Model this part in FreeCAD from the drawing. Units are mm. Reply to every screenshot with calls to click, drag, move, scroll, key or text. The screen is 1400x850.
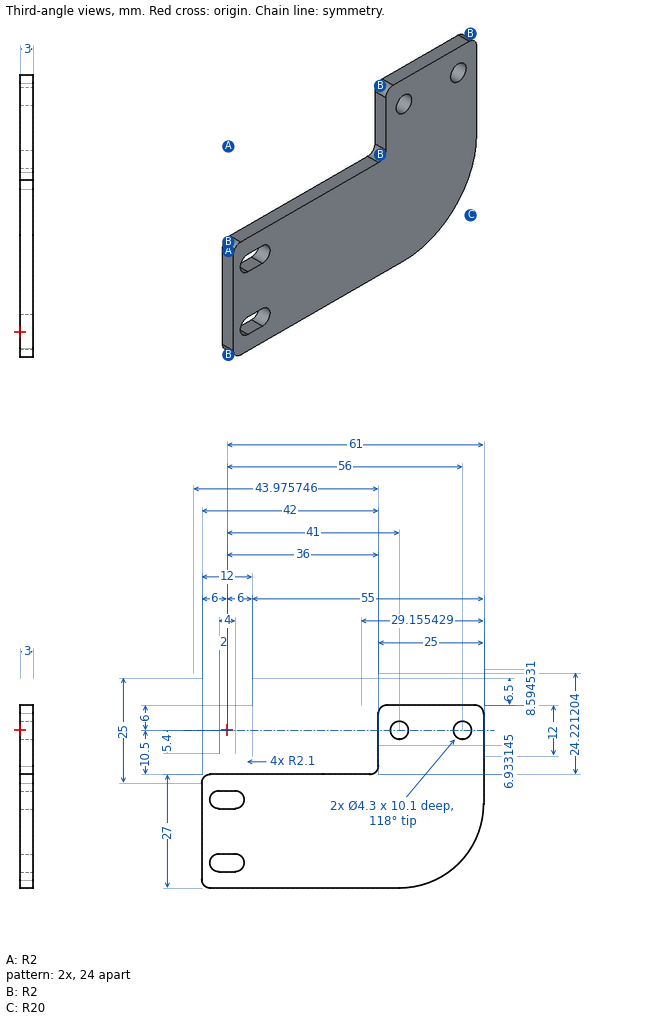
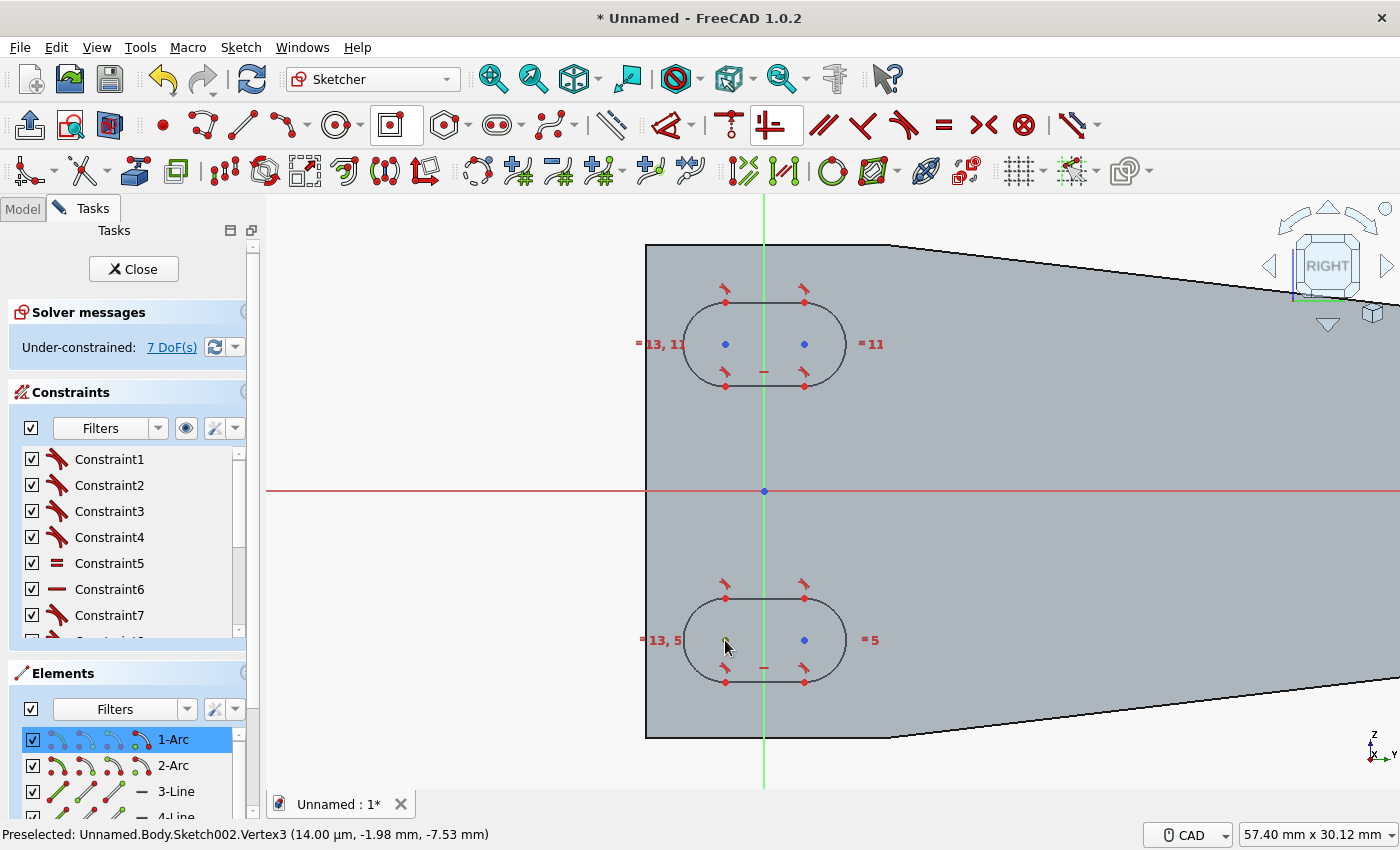
click(725, 345)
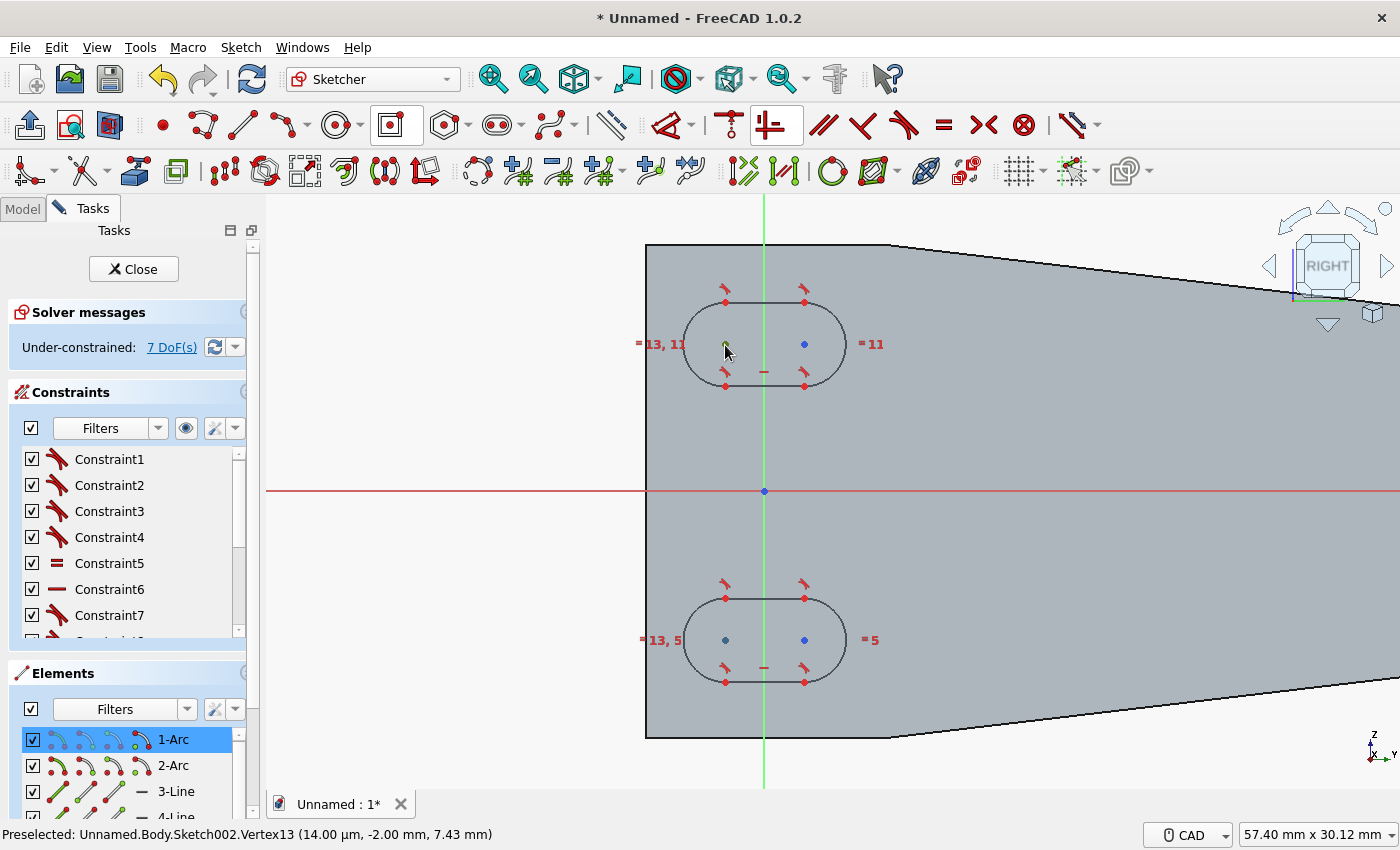
click(361, 491)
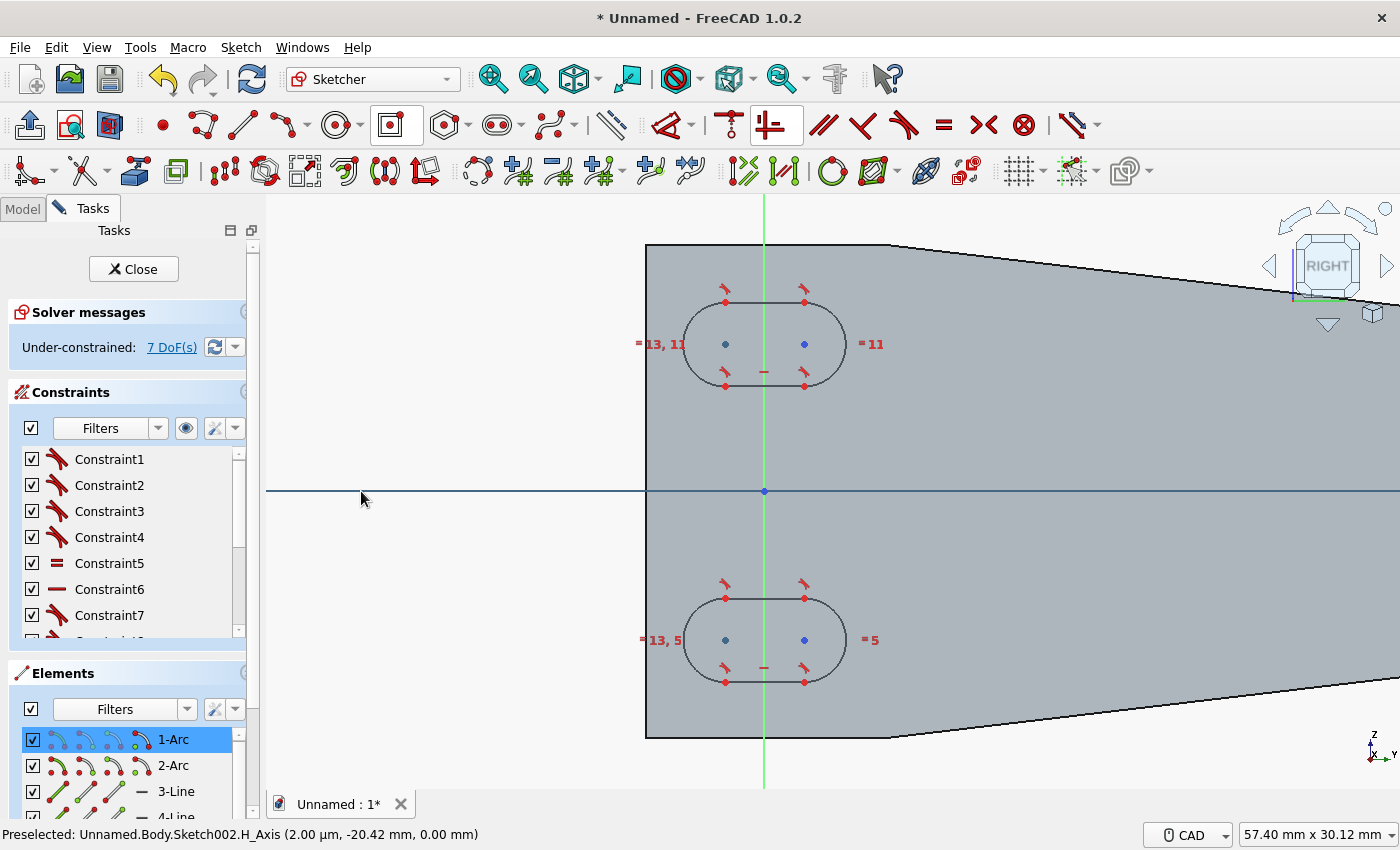
click(984, 126)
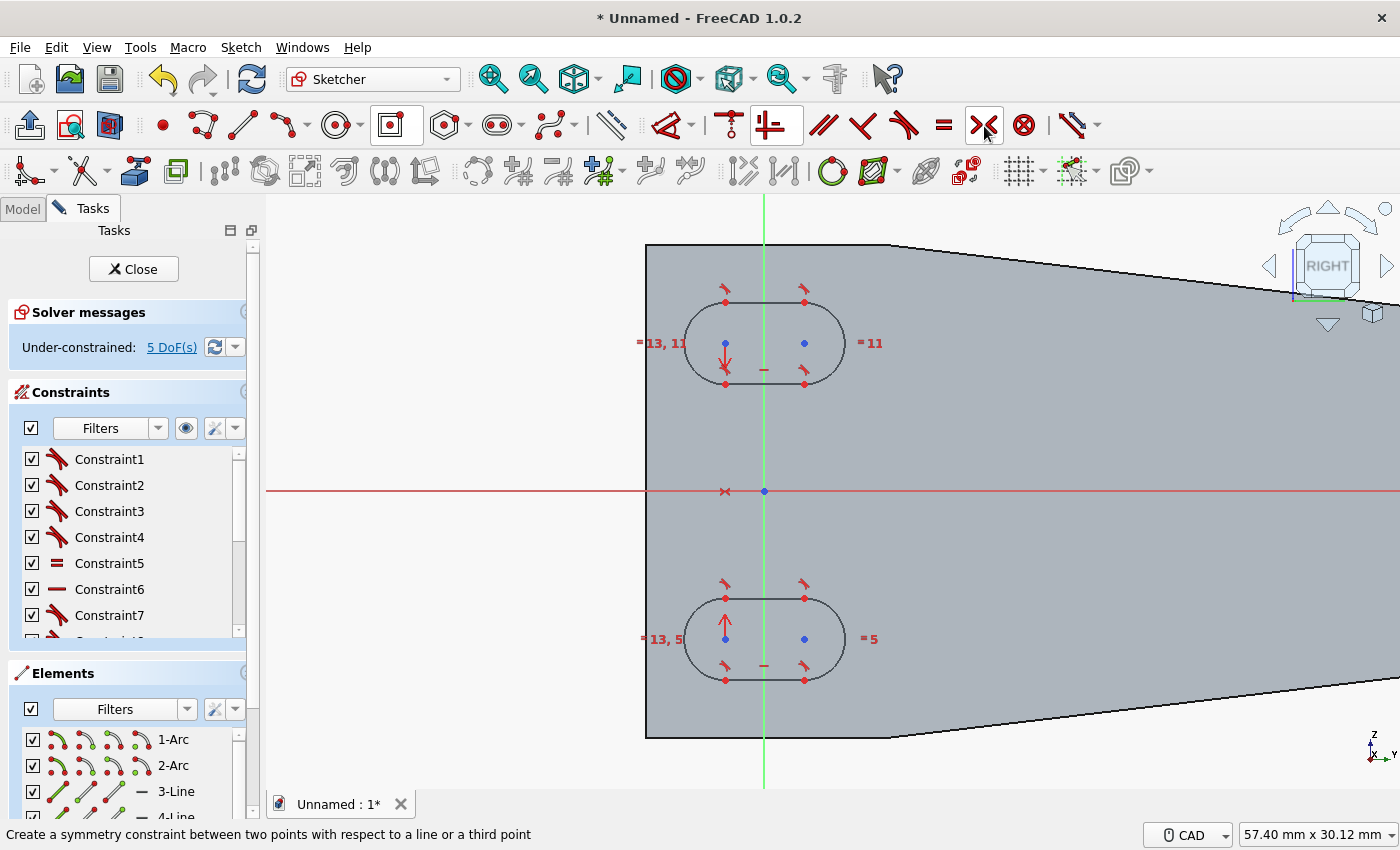
click(666, 126)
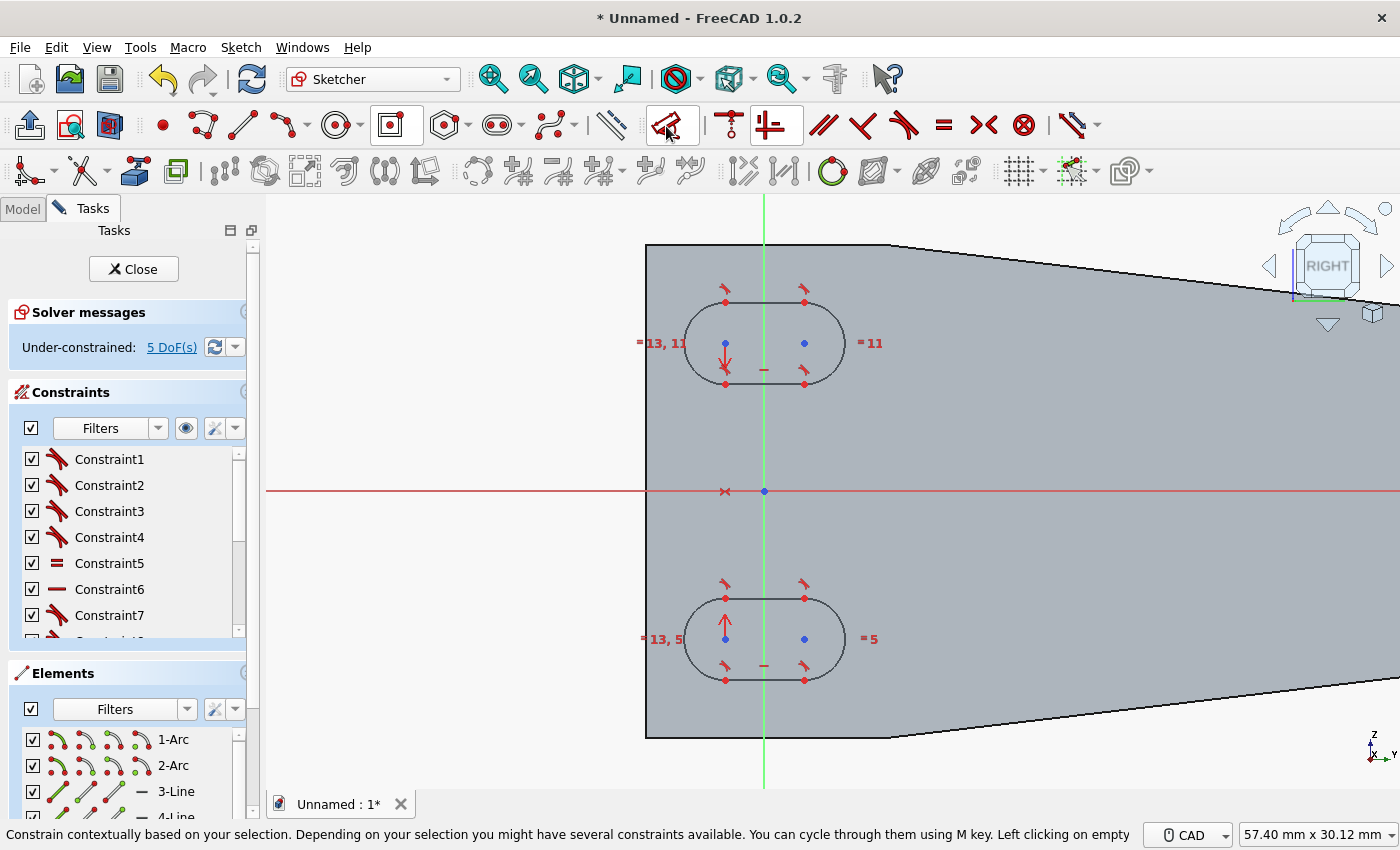
click(692, 615)
click(666, 596)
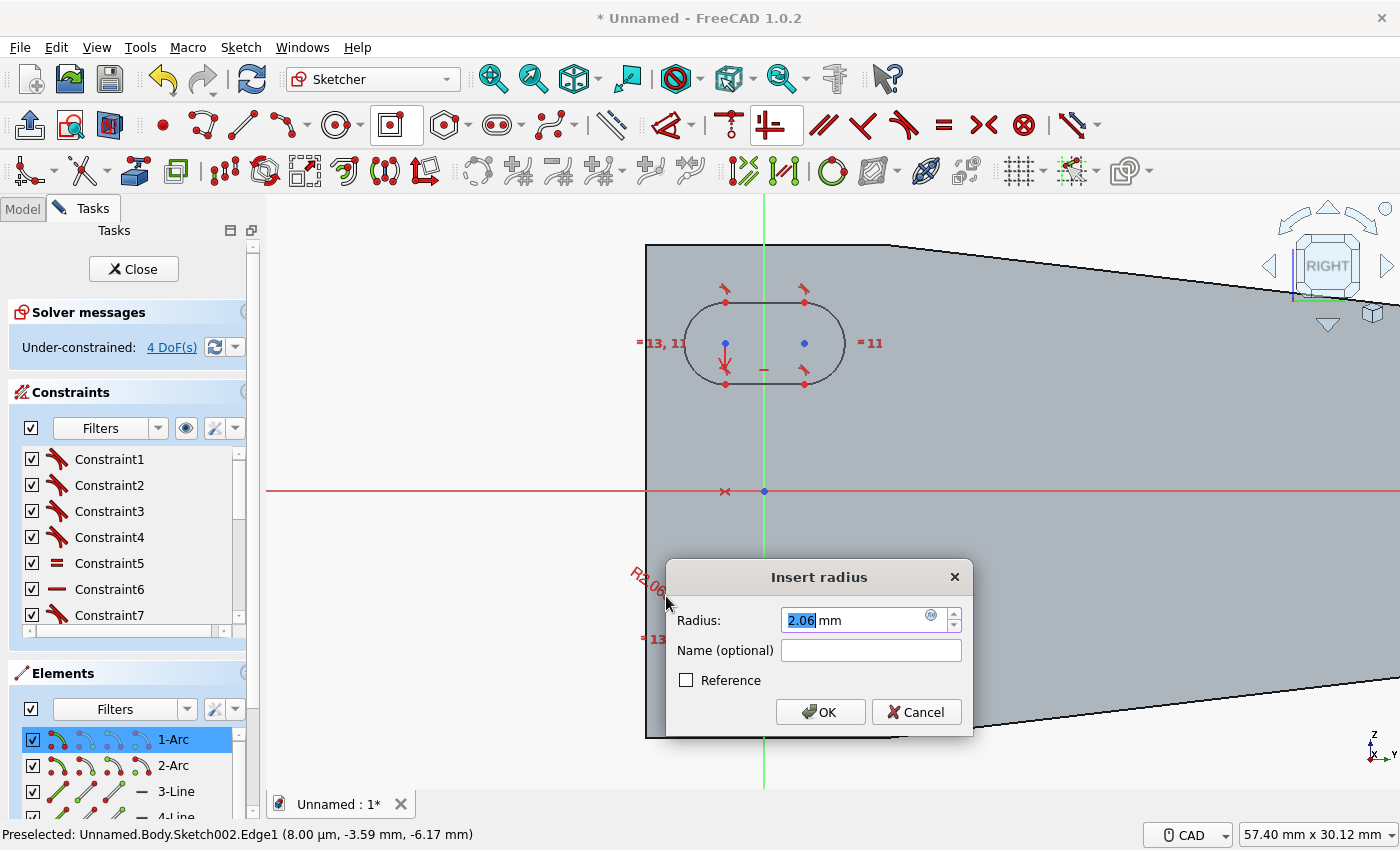
text(2.1)
key(Return)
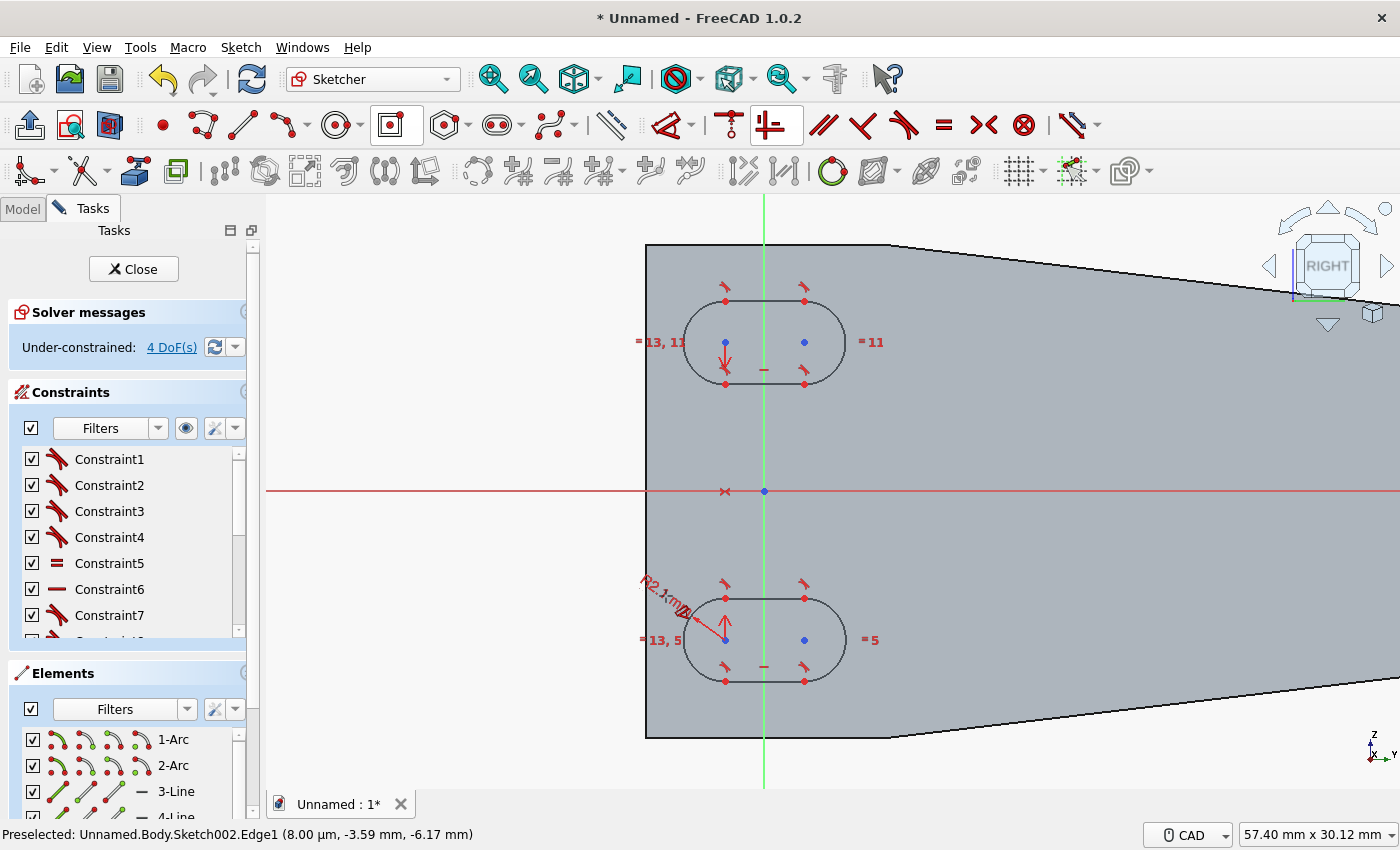
click(749, 599)
click(746, 633)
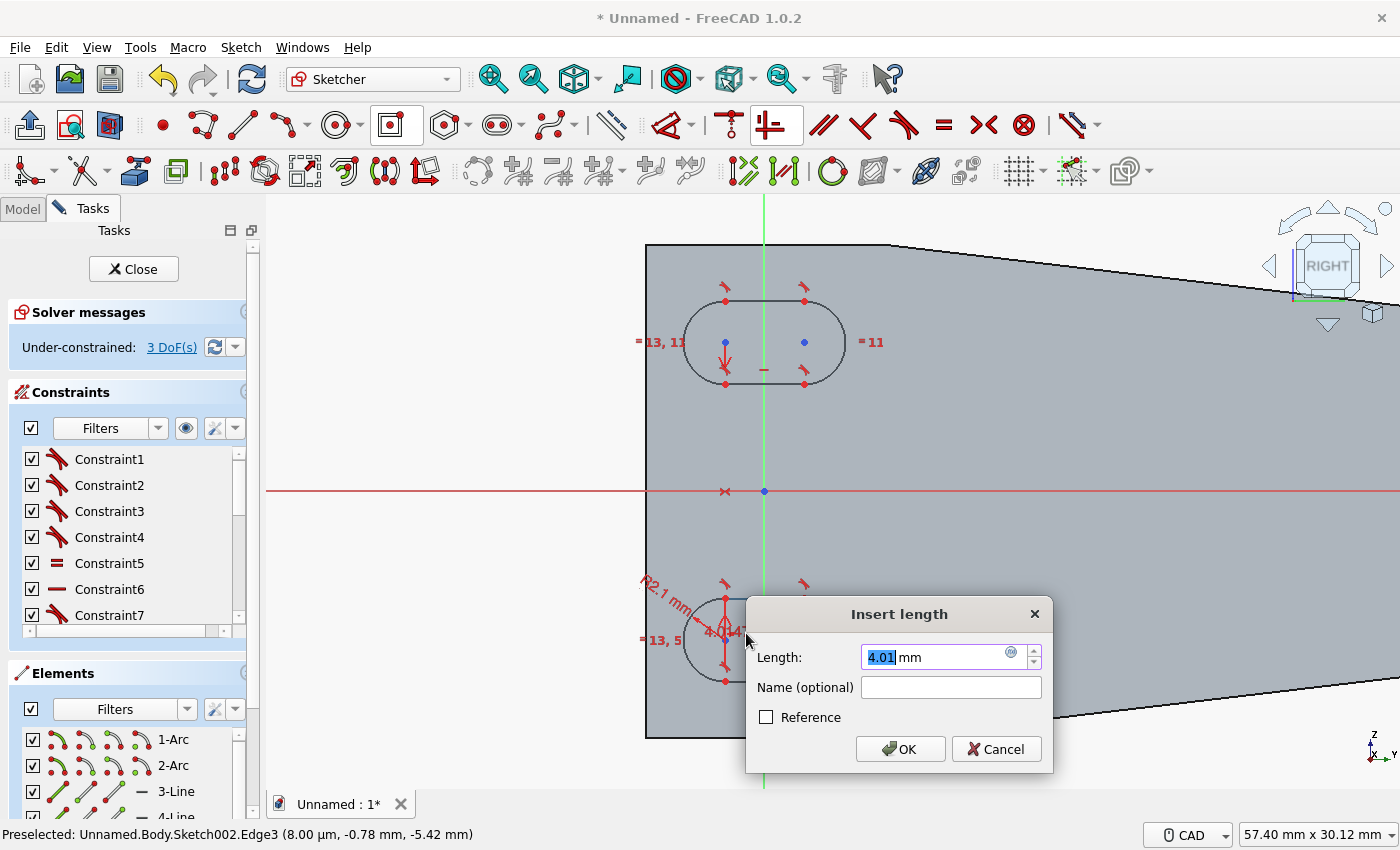
text(4)
key(Return)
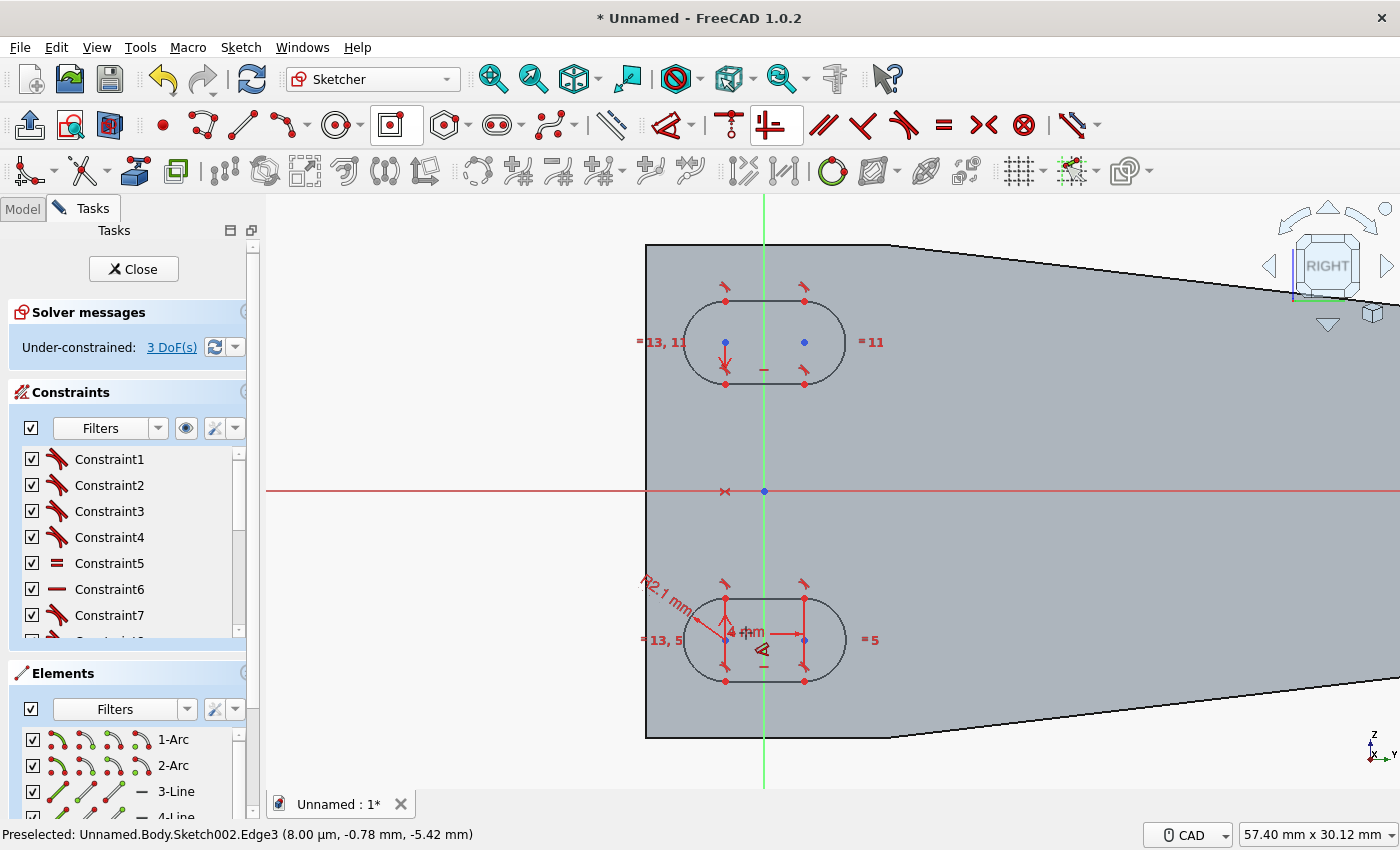
click(749, 301)
click(747, 267)